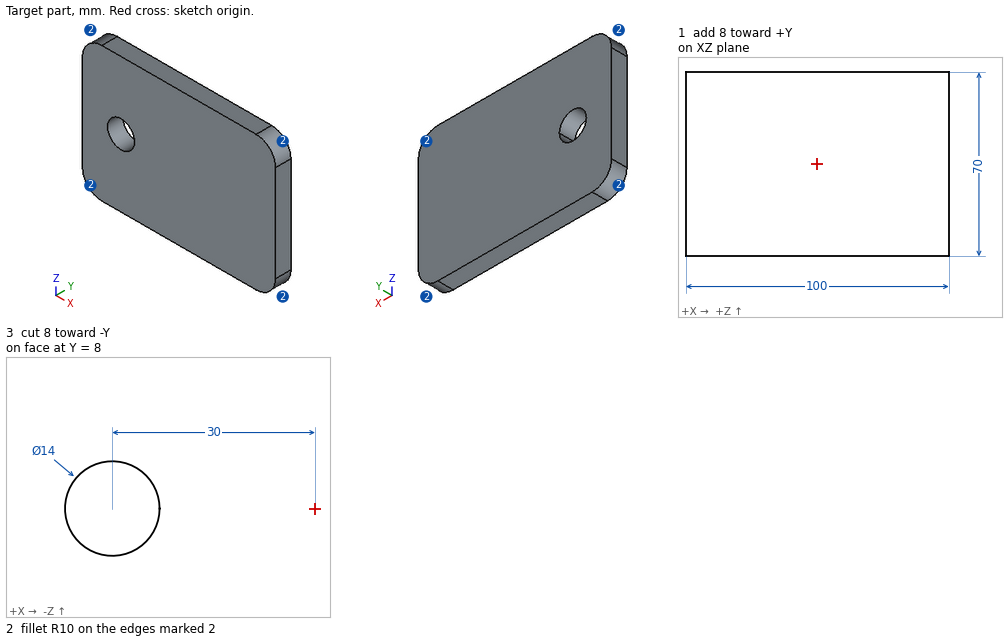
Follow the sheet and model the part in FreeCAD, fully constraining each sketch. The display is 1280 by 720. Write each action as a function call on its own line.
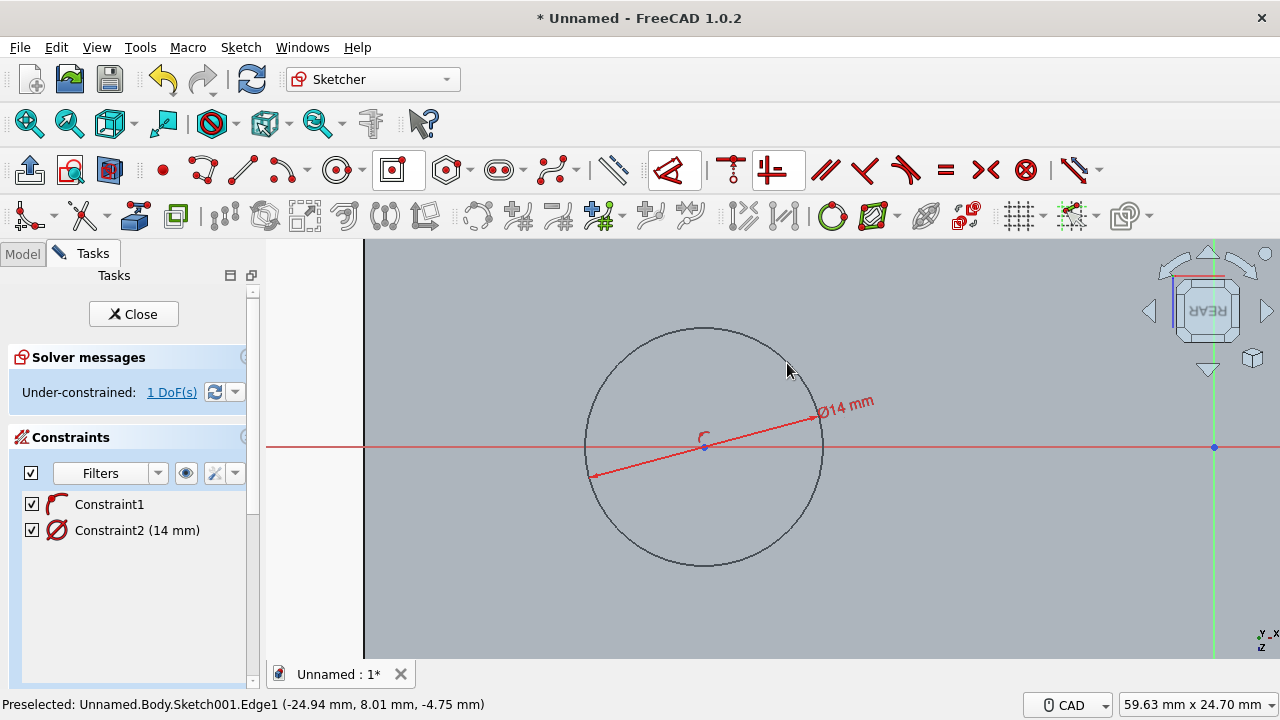
click(704, 447)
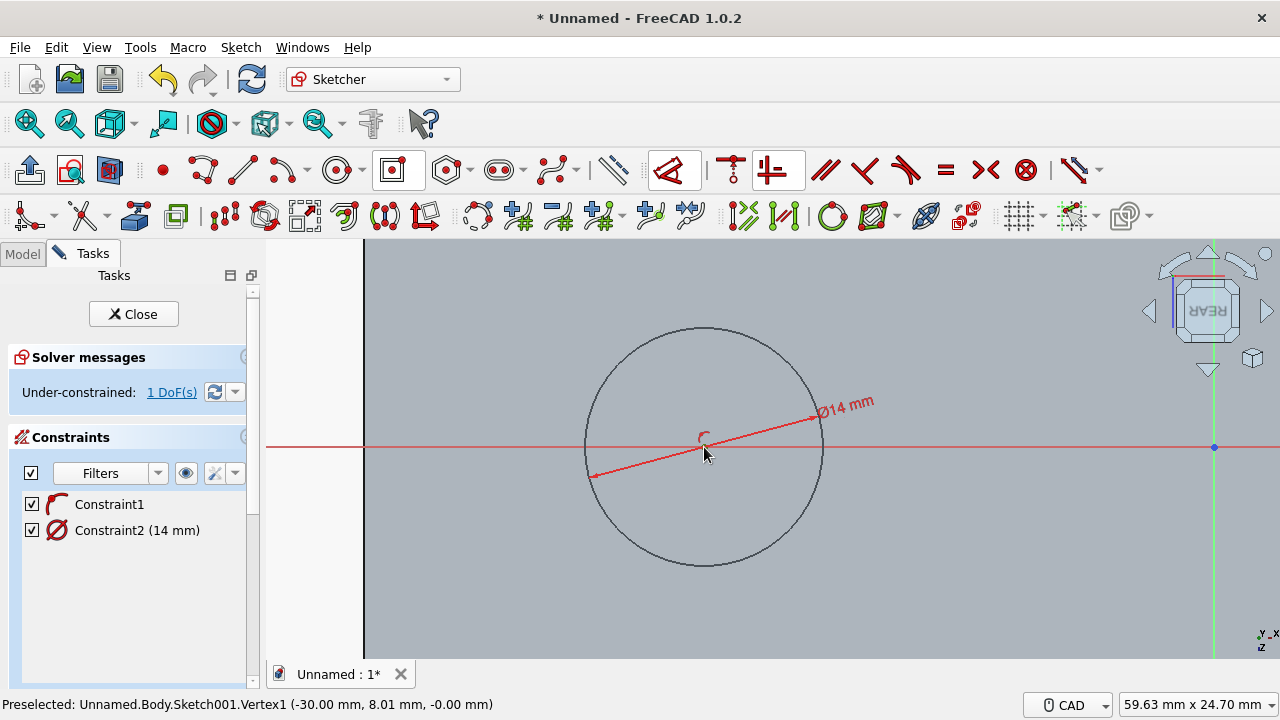
click(696, 170)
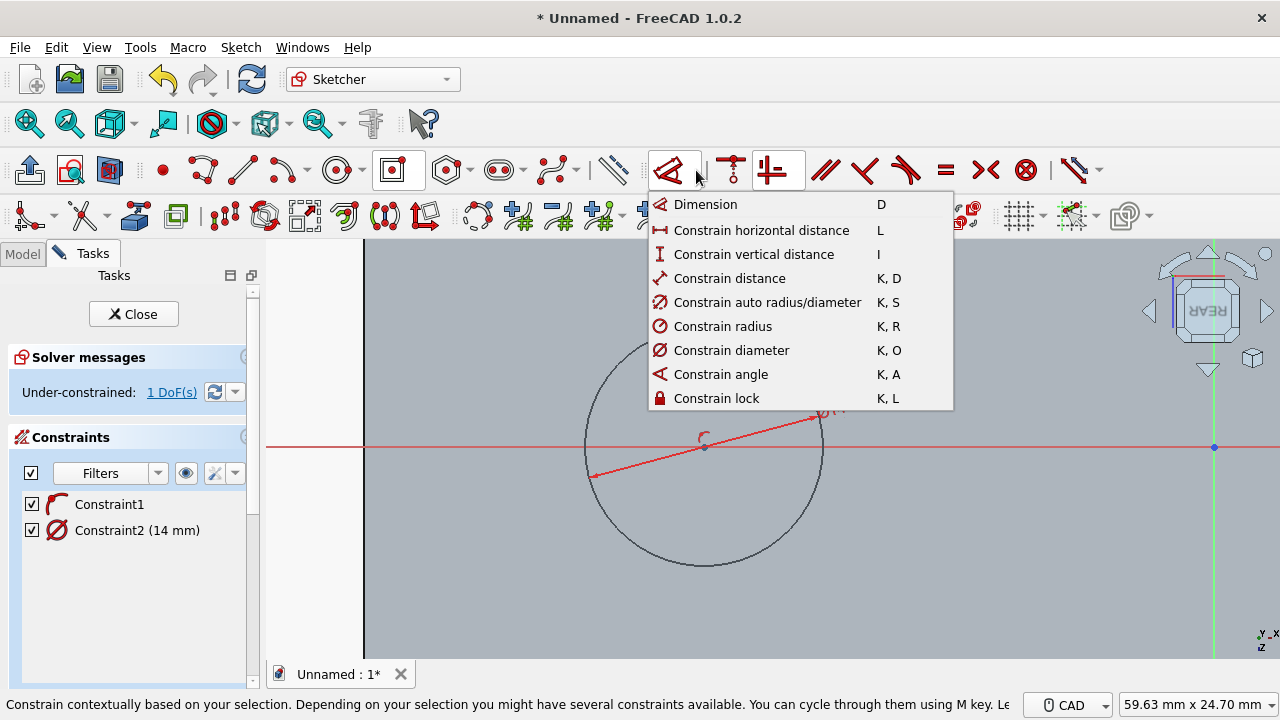
click(801, 230)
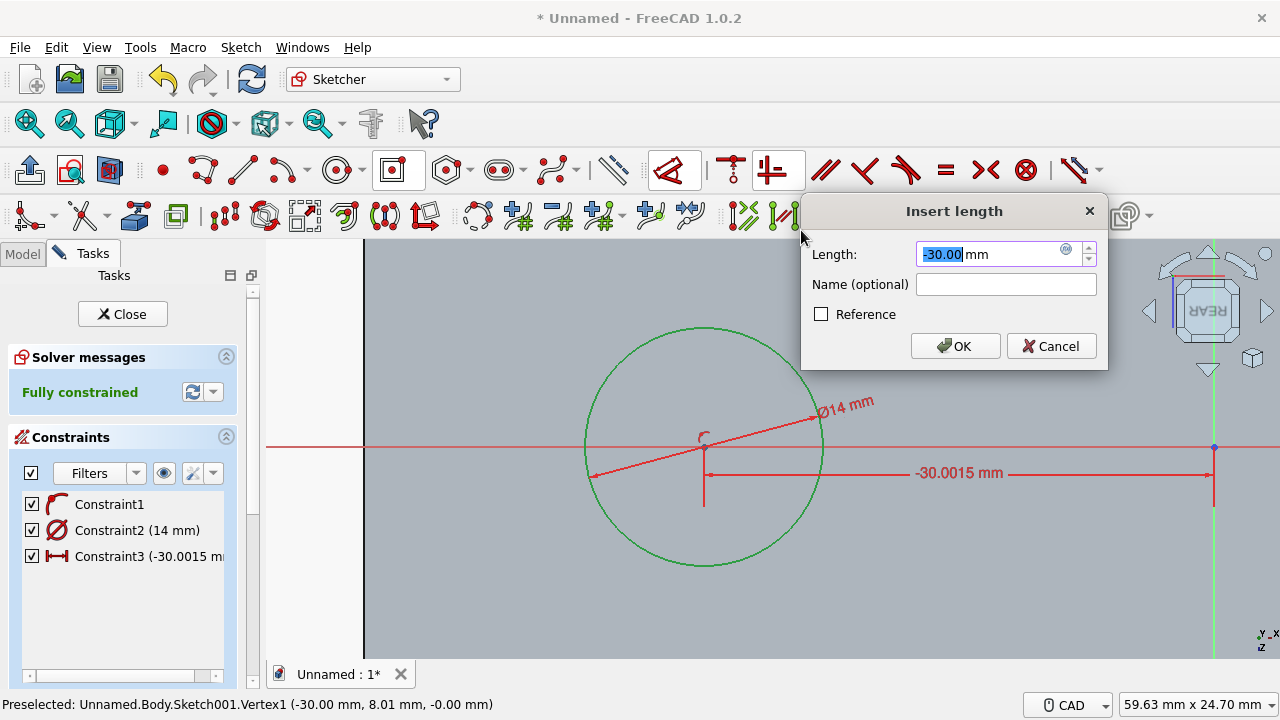
text(-30)
key(Return)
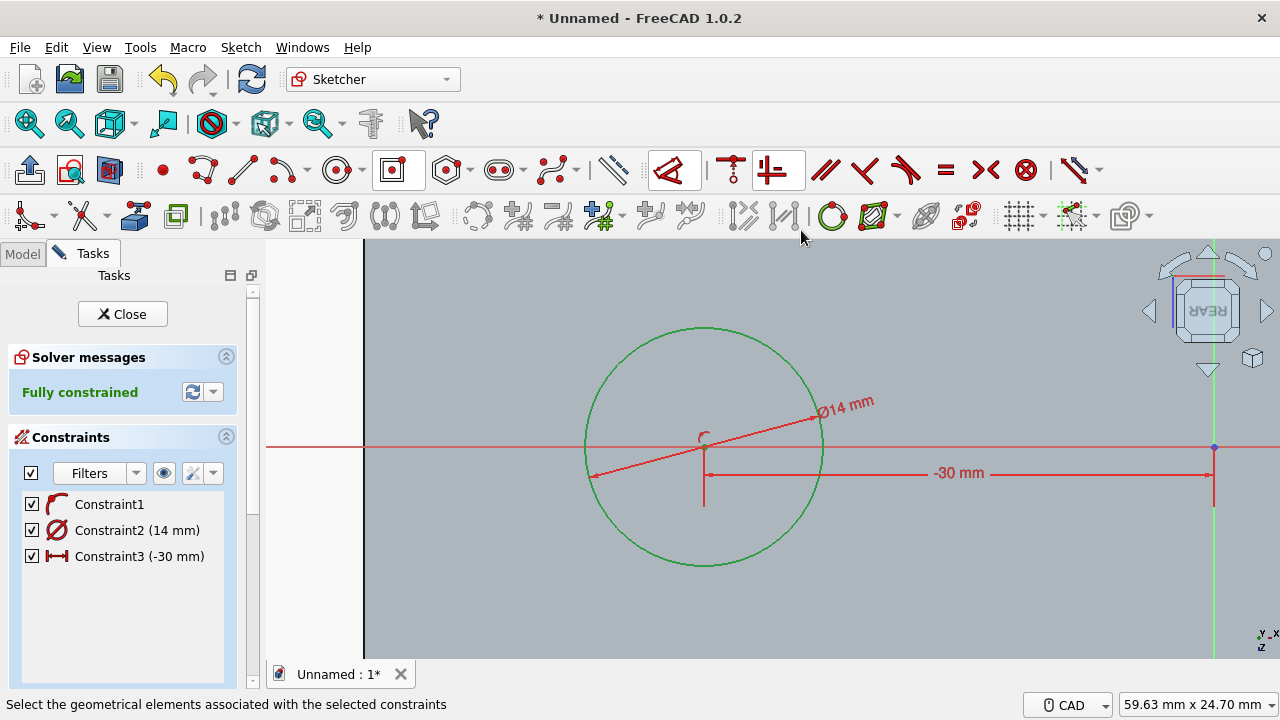
click(123, 314)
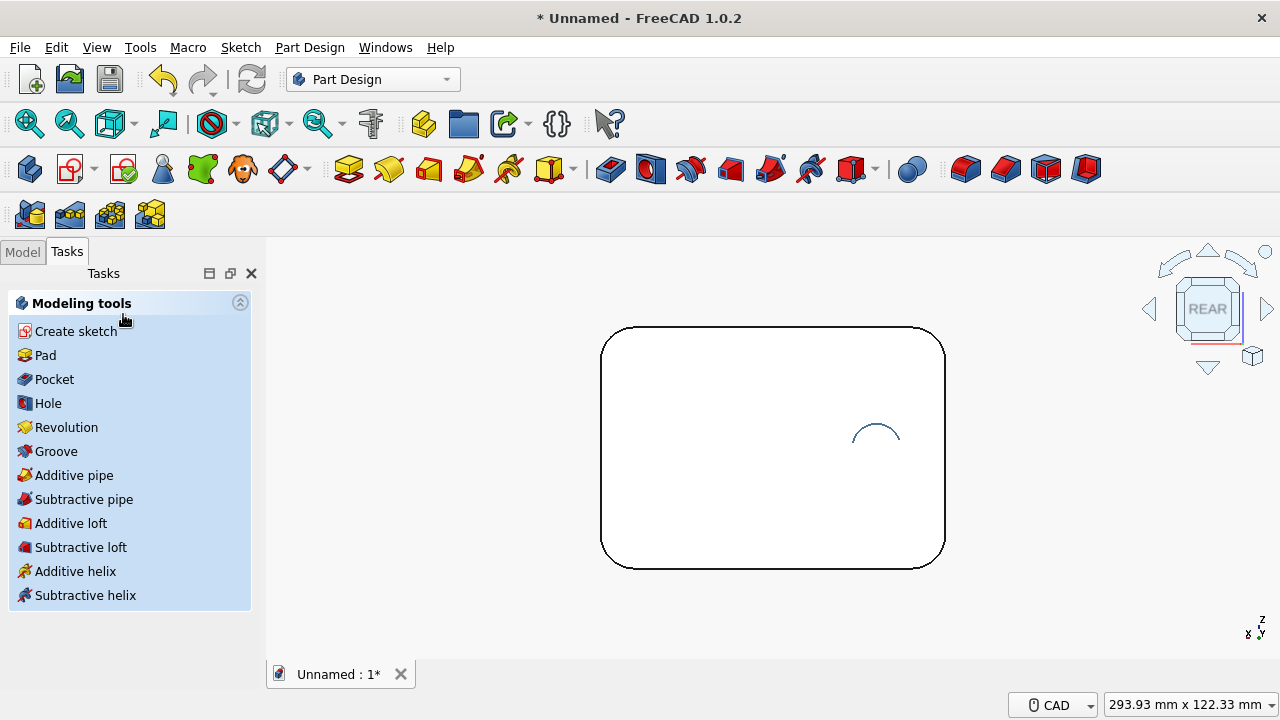
click(612, 170)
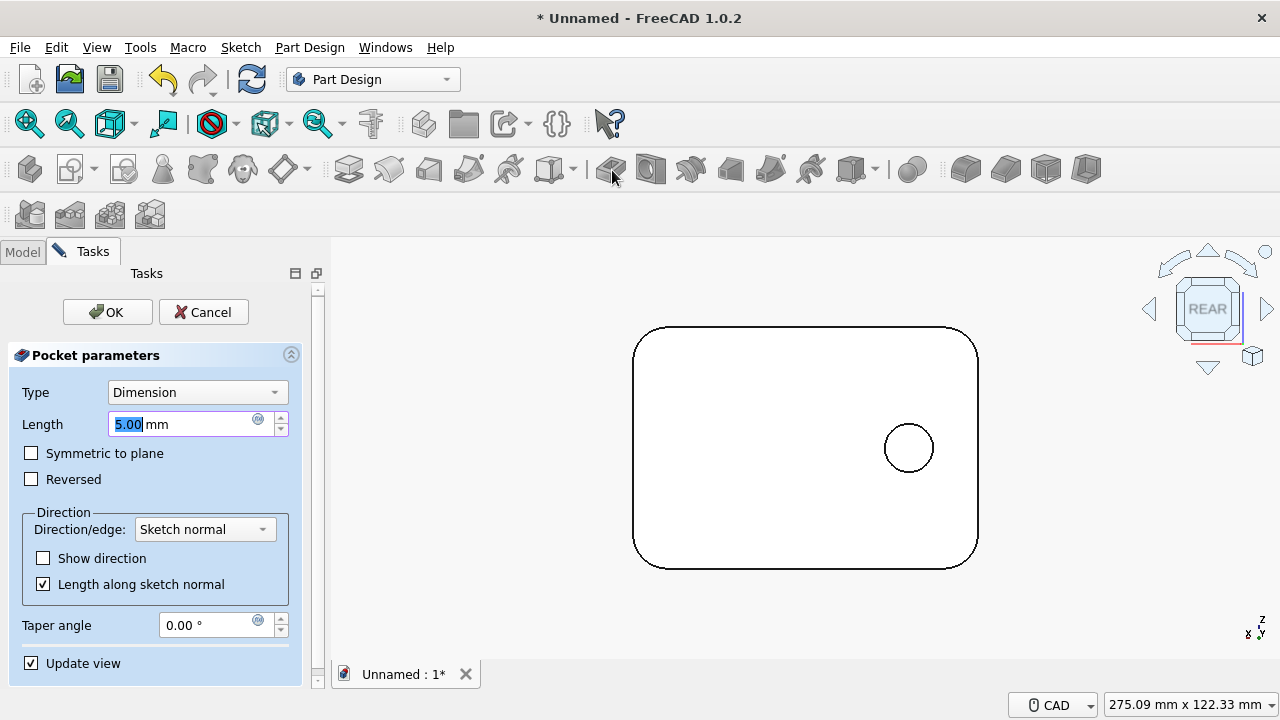
text(8)
key(Tab)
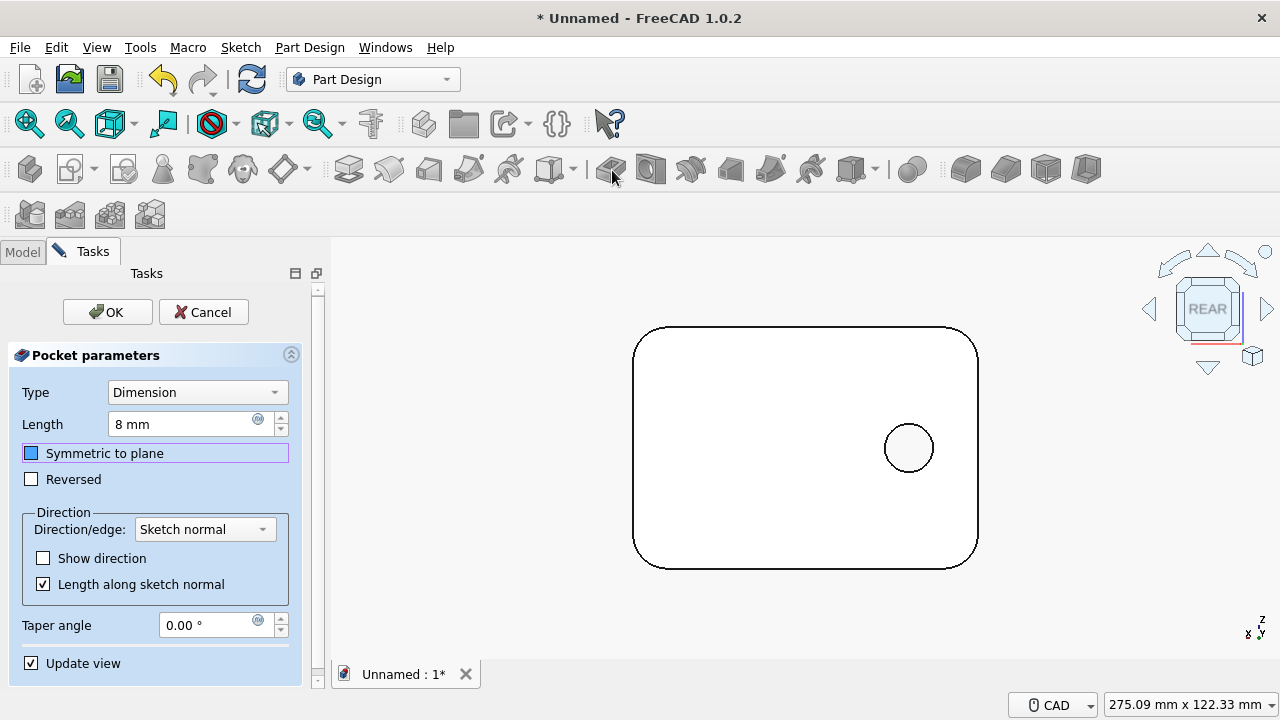
click(108, 312)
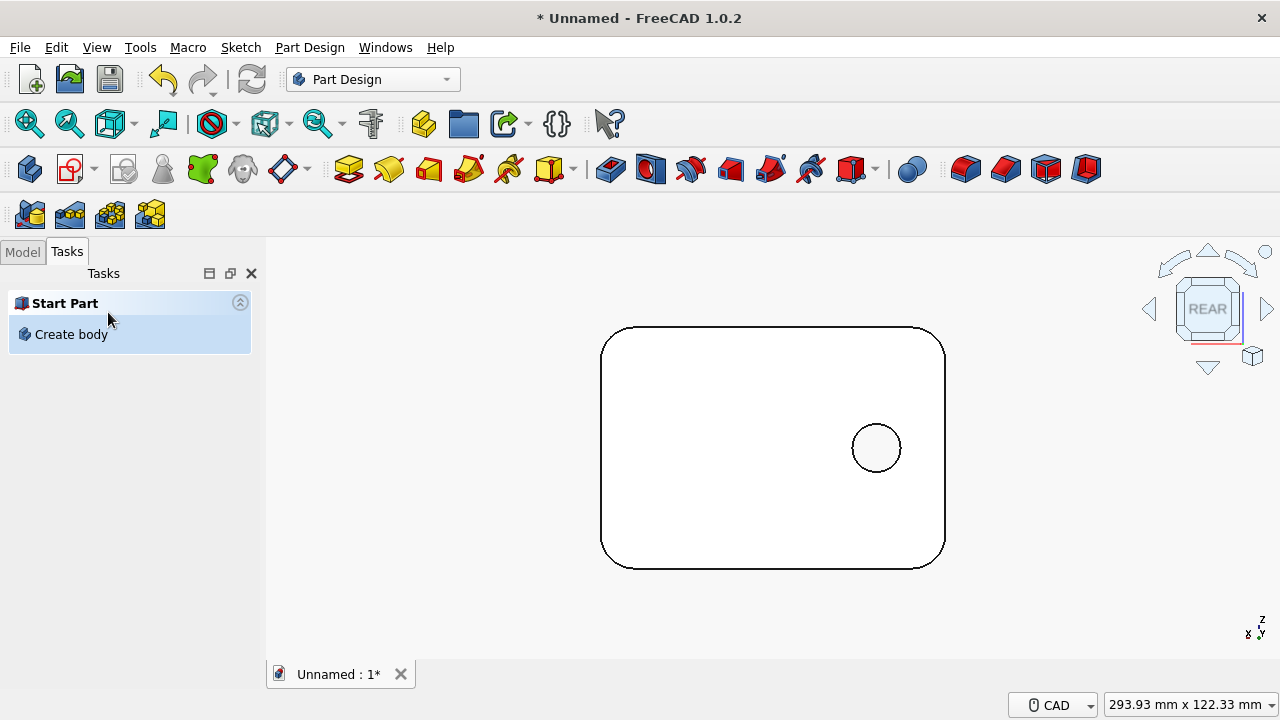
key(0)